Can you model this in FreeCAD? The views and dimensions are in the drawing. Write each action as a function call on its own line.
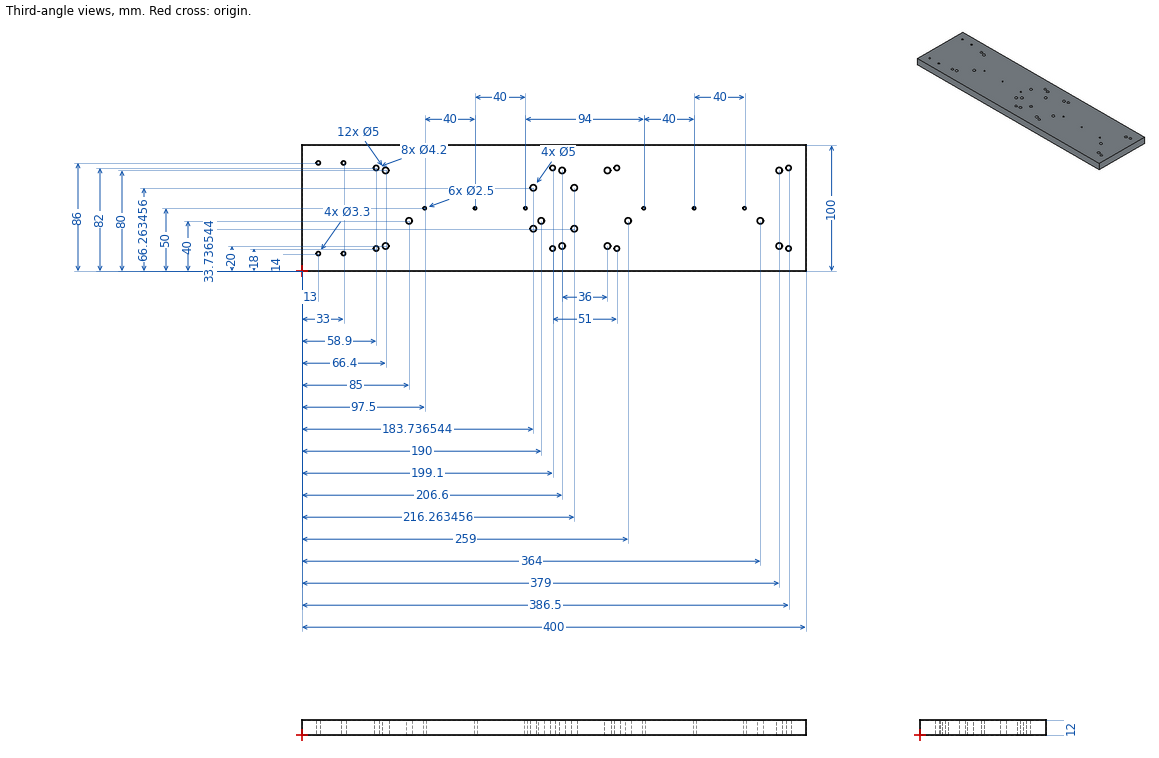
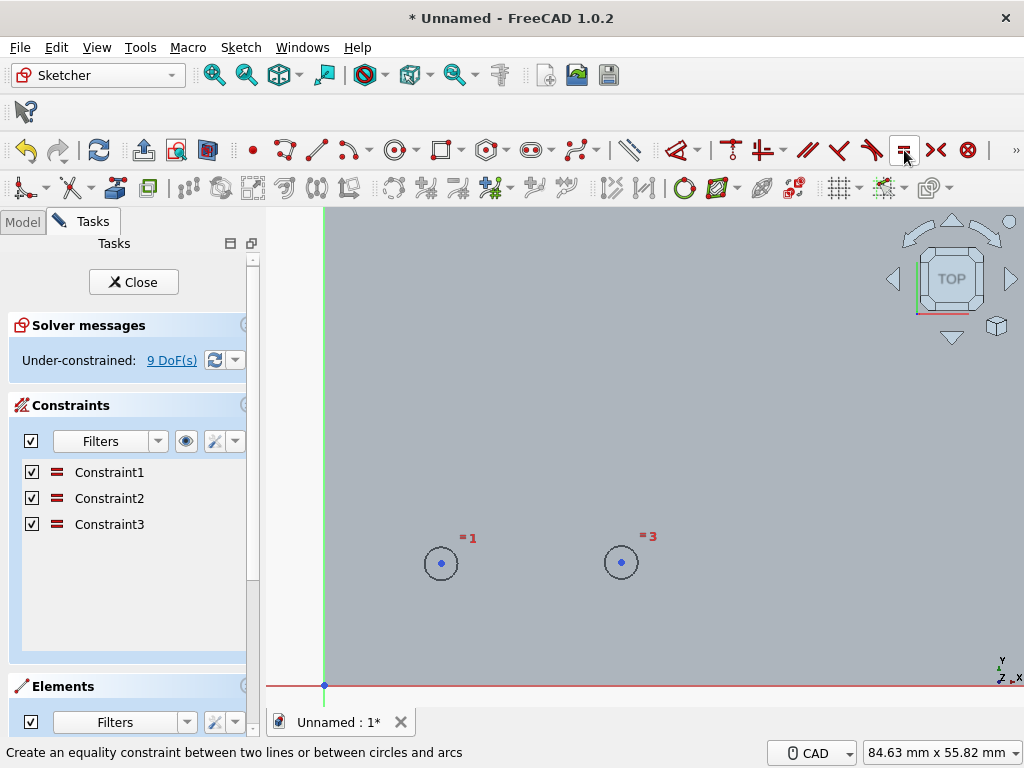
click(441, 564)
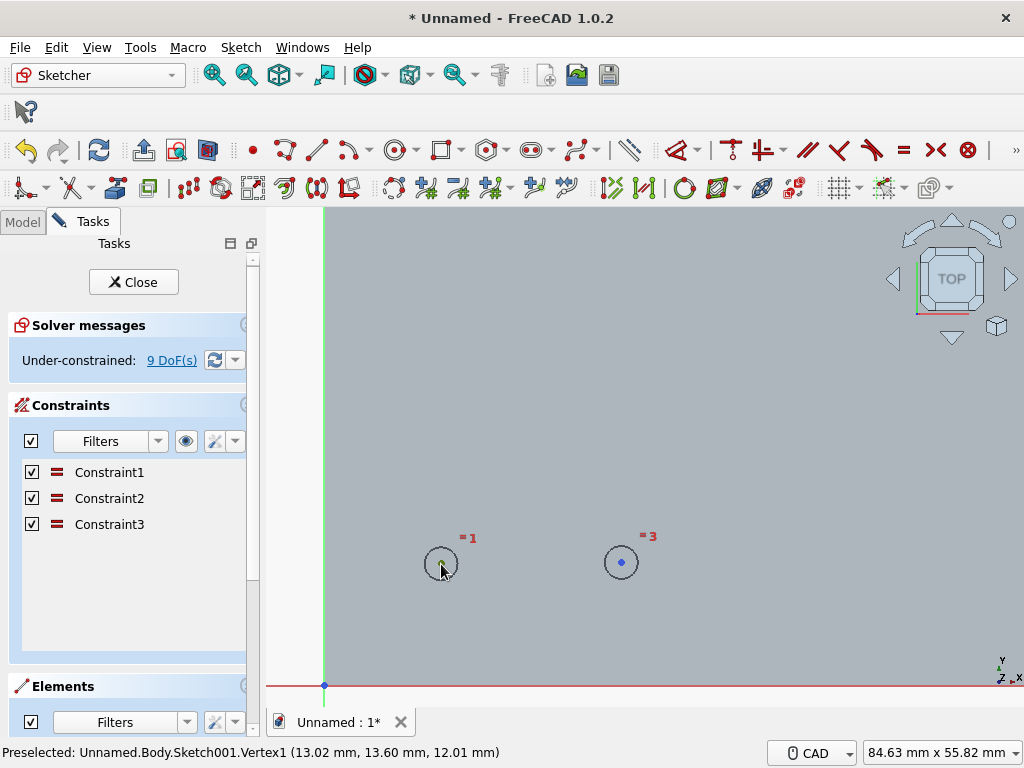
scroll(633, 552, down, 5)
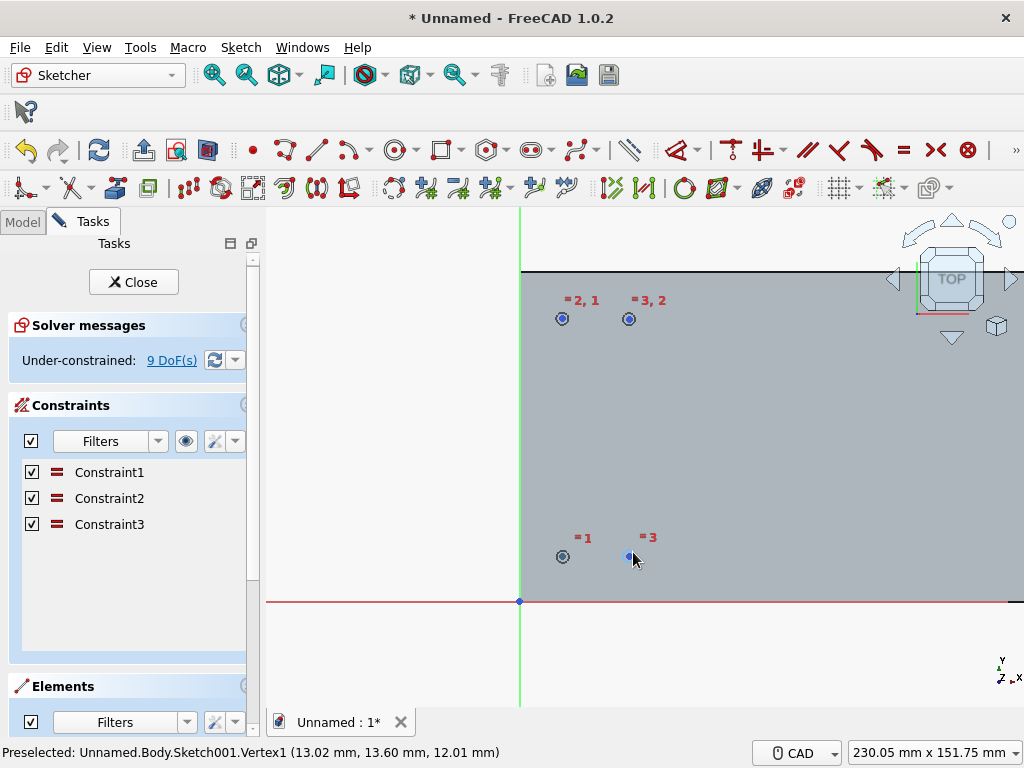
click(562, 319)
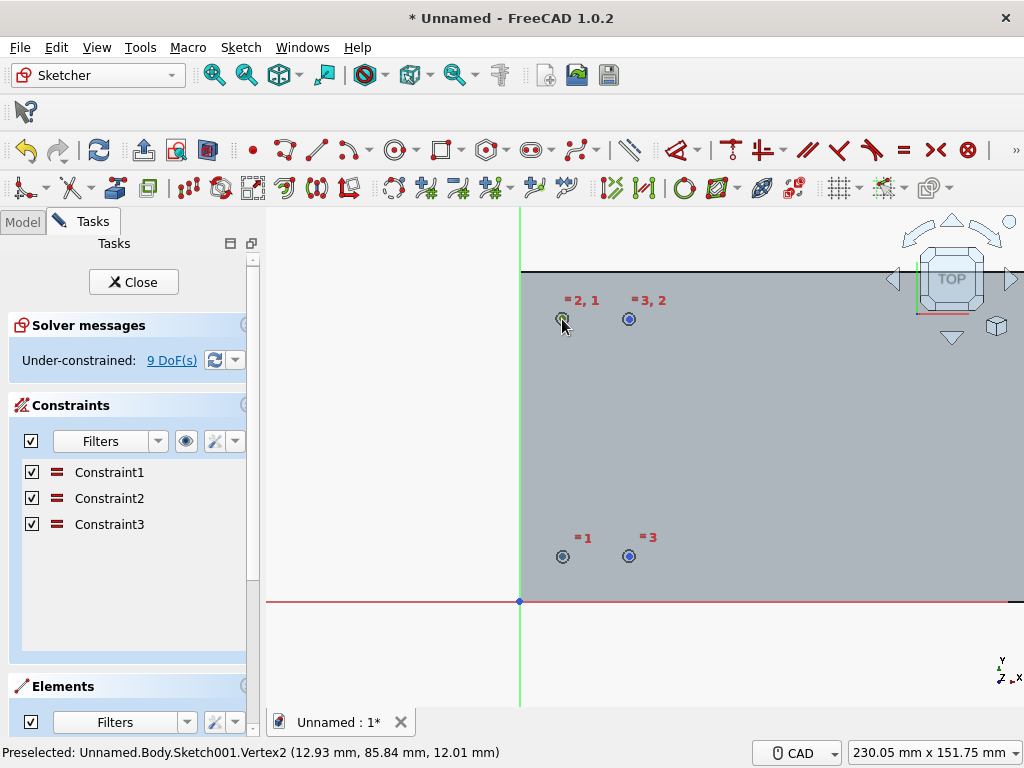
key(v)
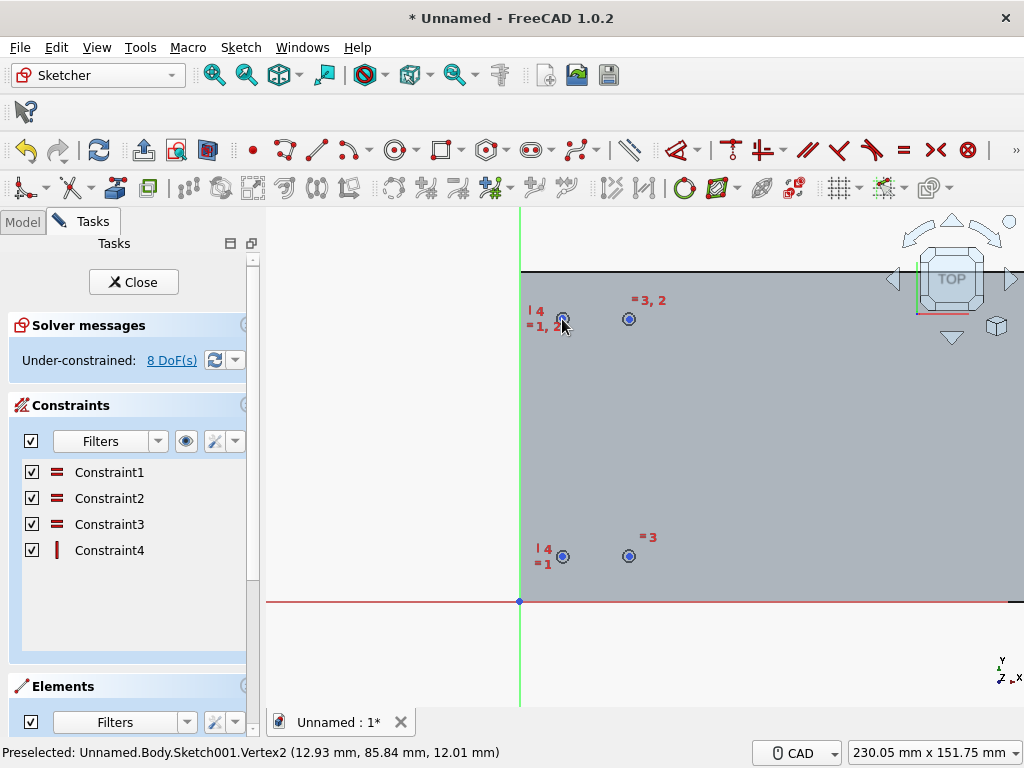
click(563, 319)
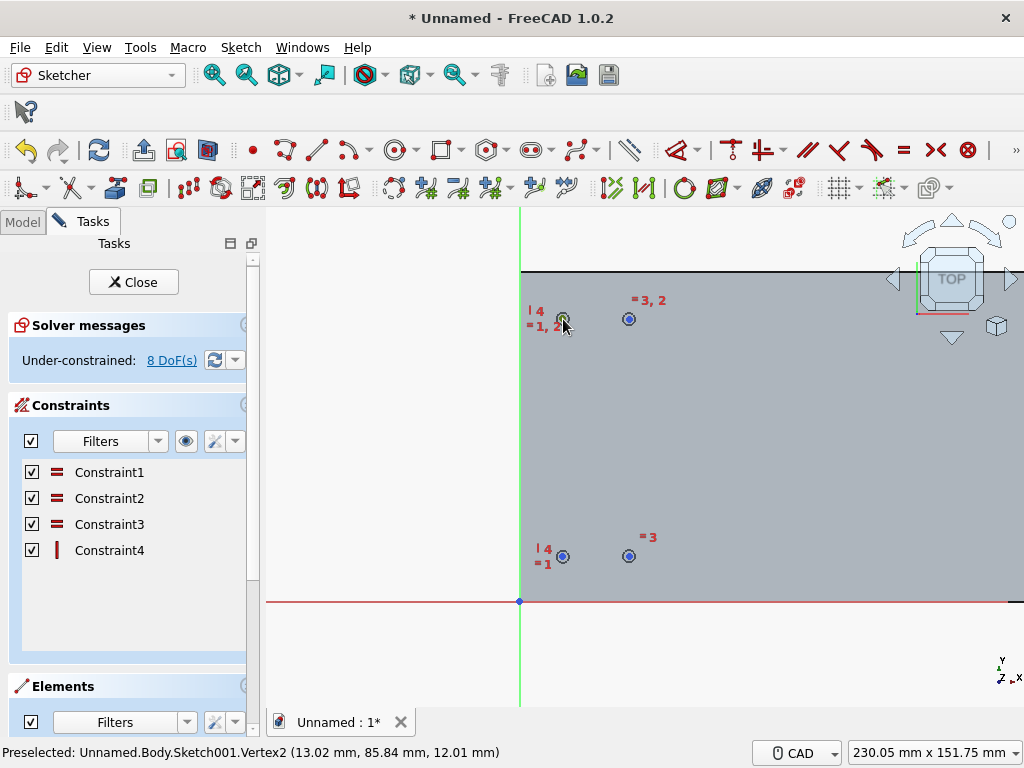
click(629, 319)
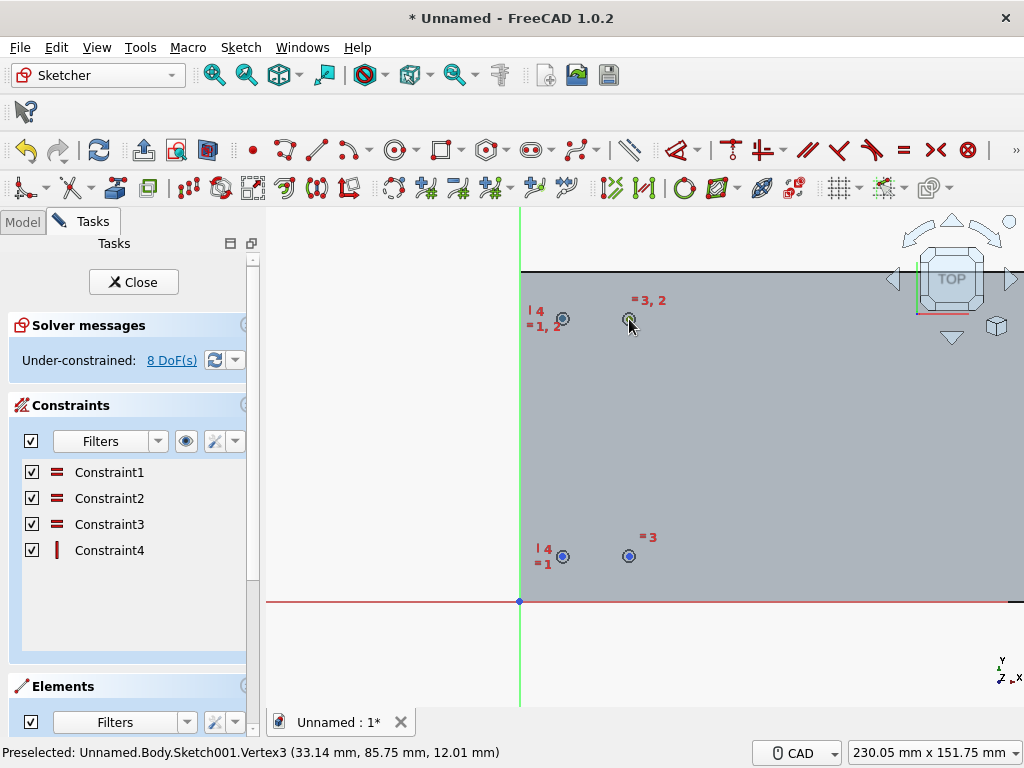
click(786, 150)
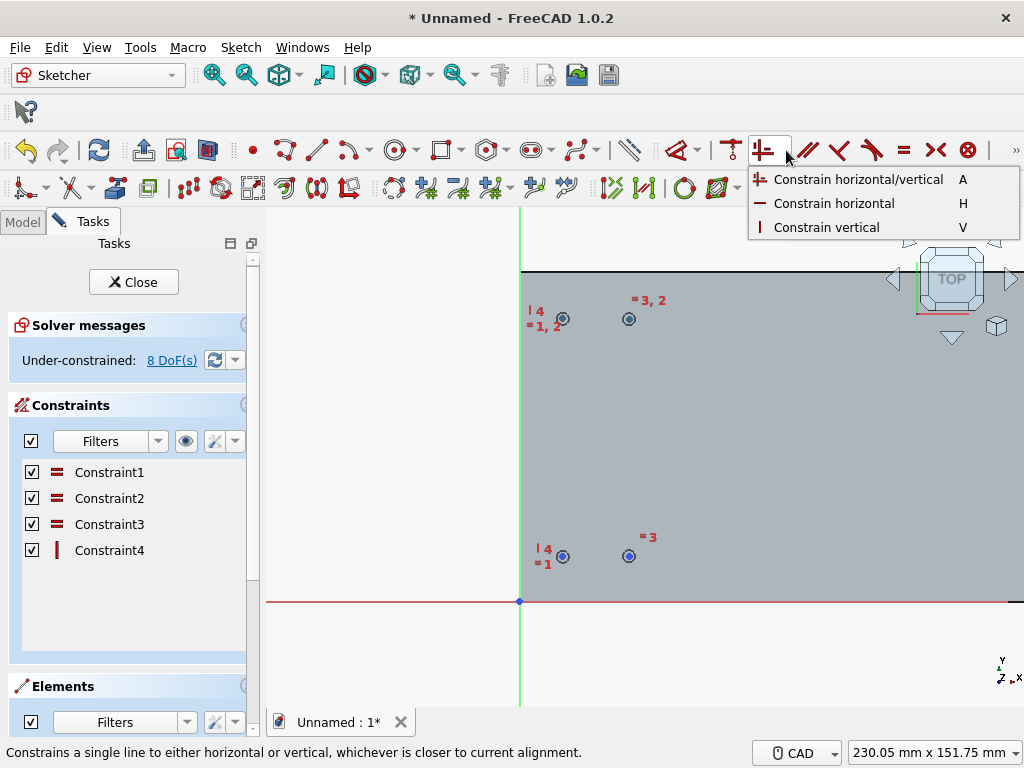
click(884, 203)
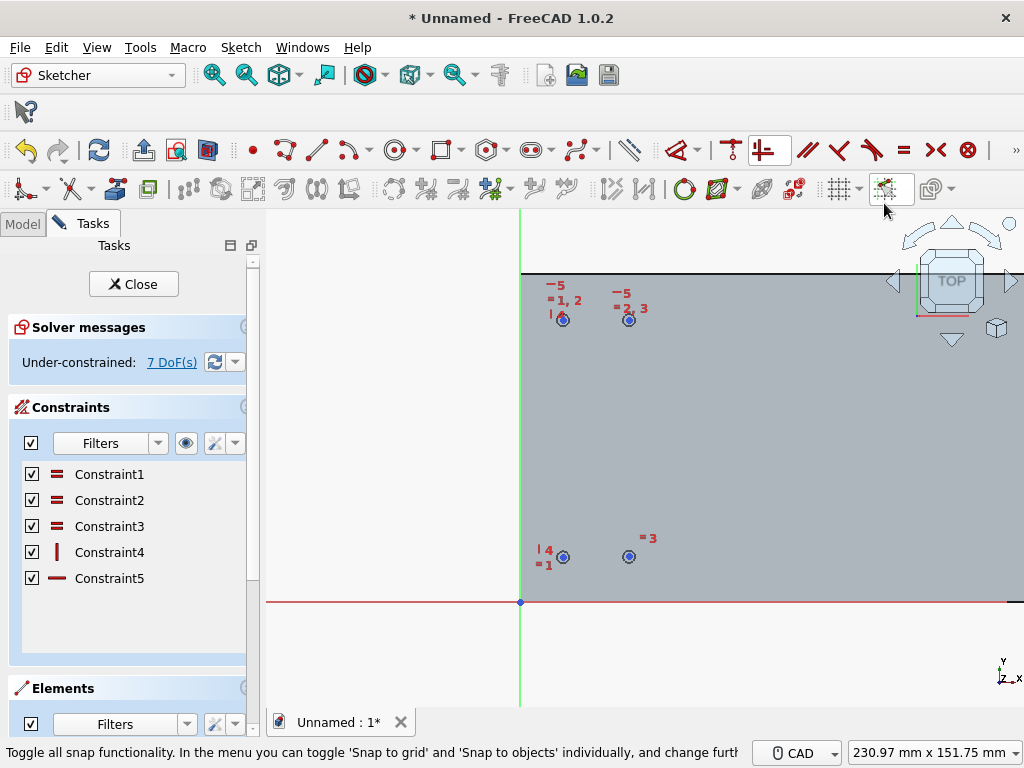
click(629, 320)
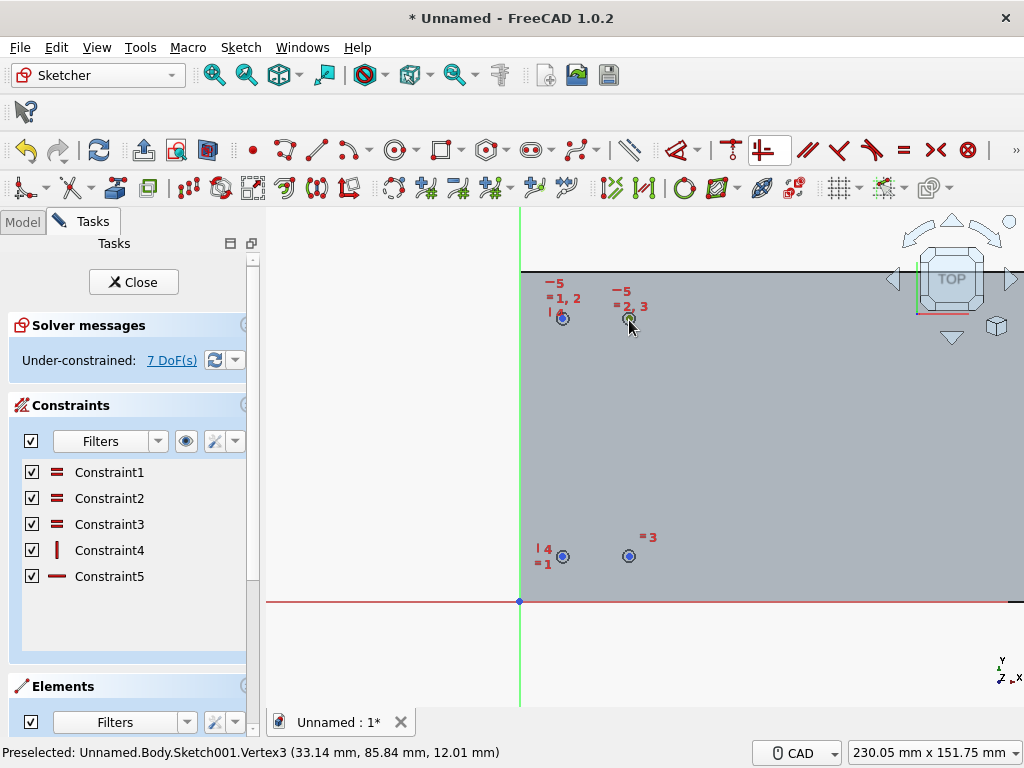
click(629, 556)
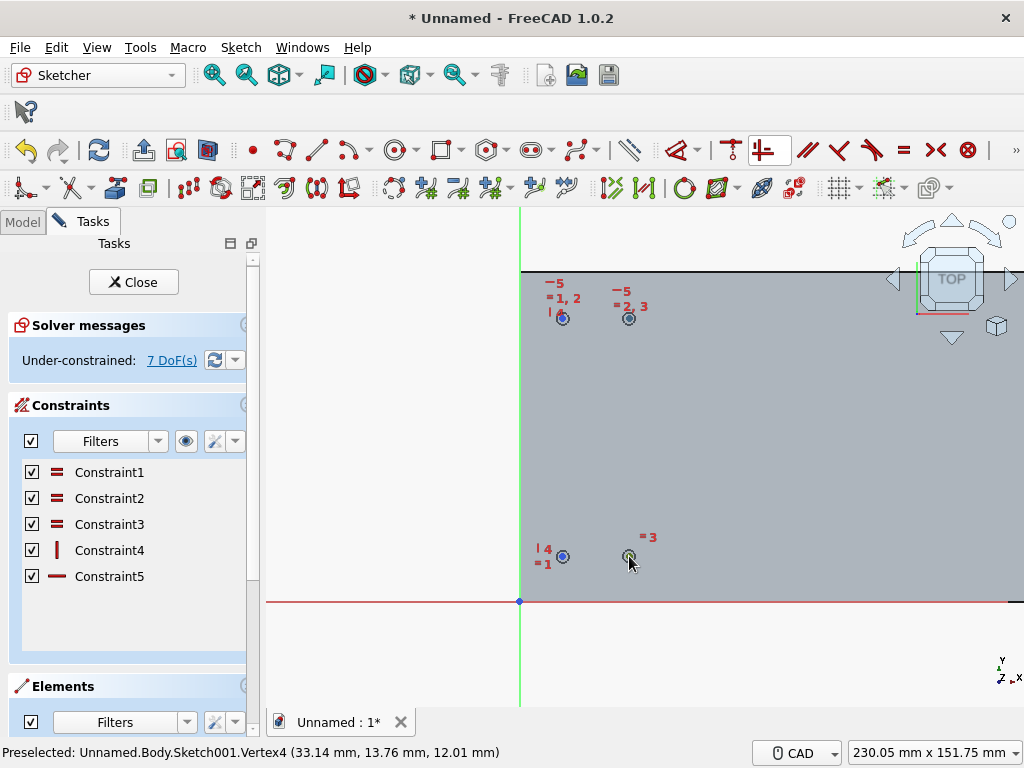
click(786, 150)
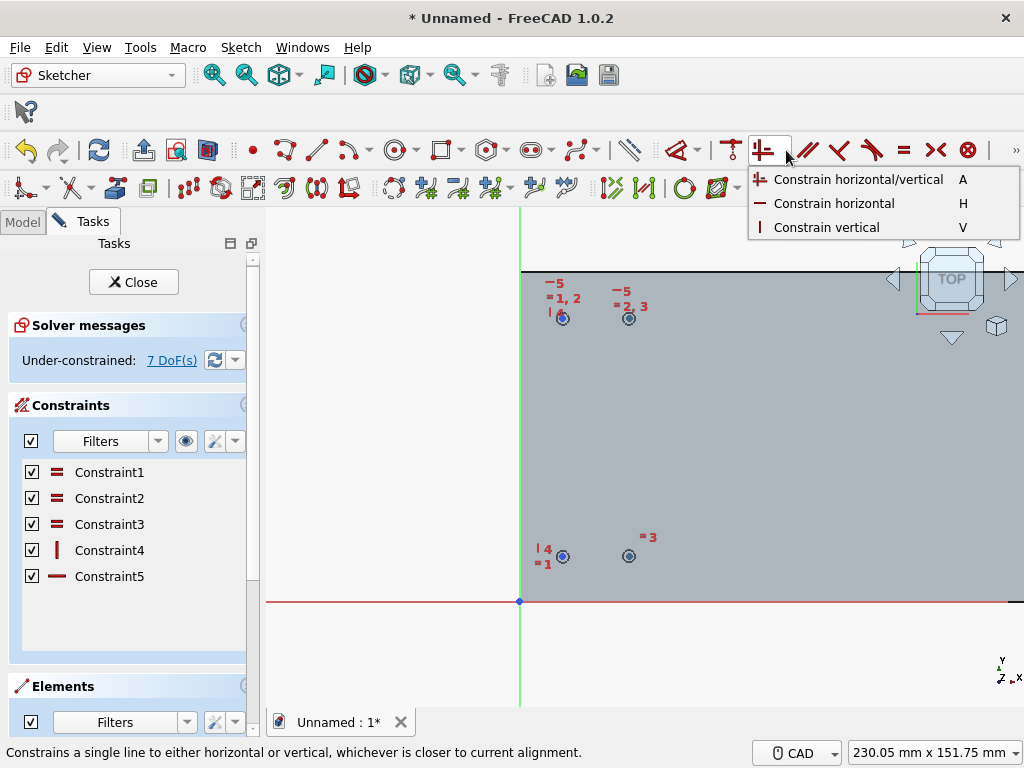
click(884, 227)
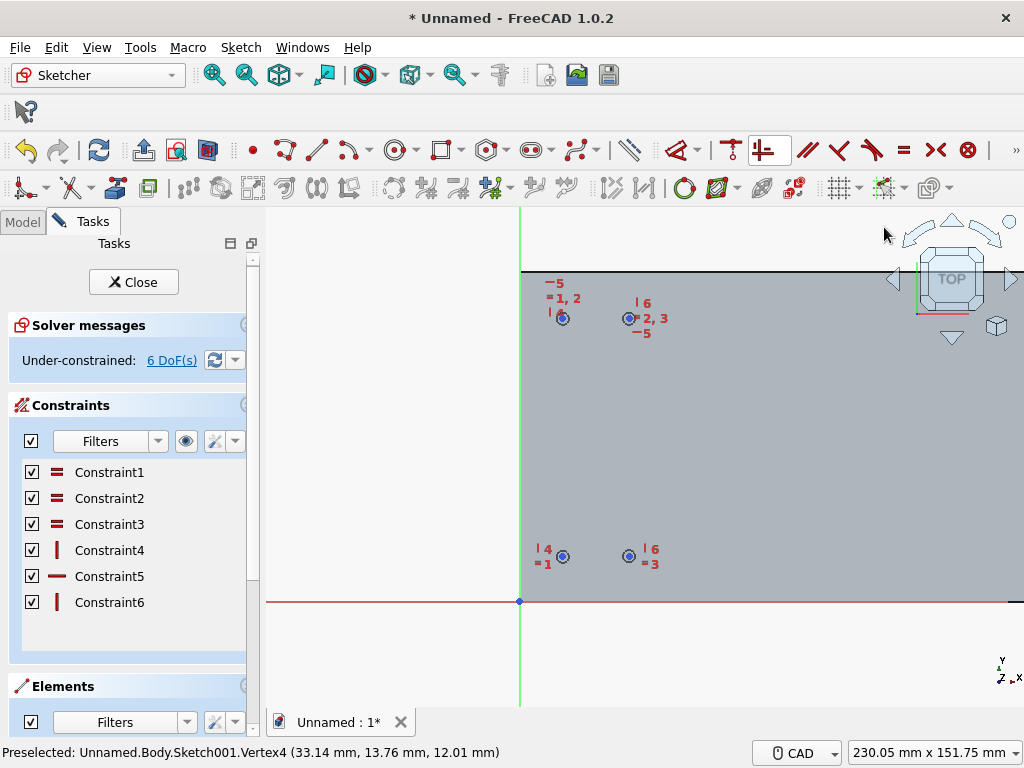
click(563, 557)